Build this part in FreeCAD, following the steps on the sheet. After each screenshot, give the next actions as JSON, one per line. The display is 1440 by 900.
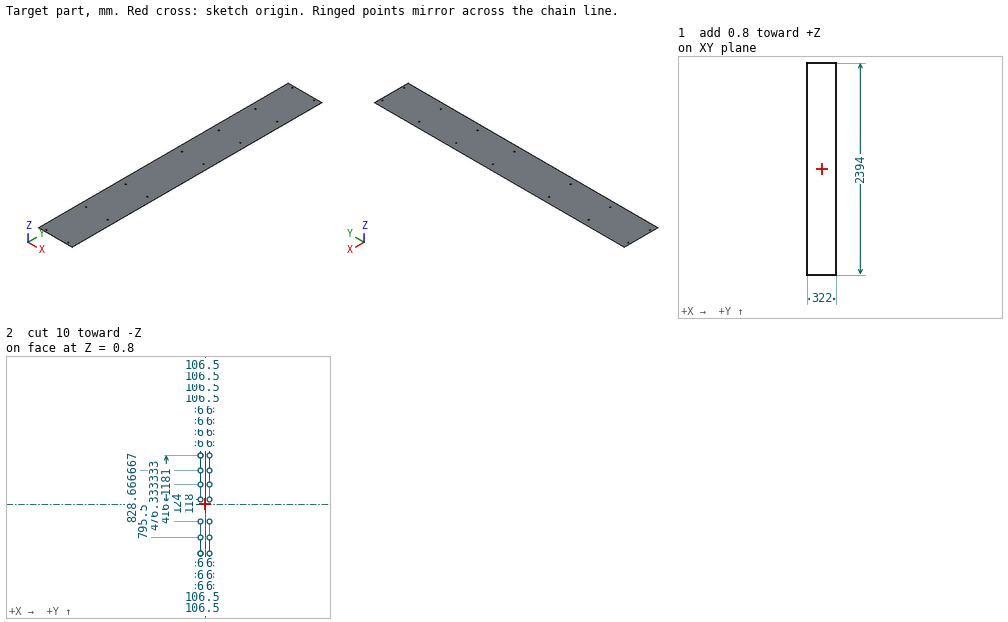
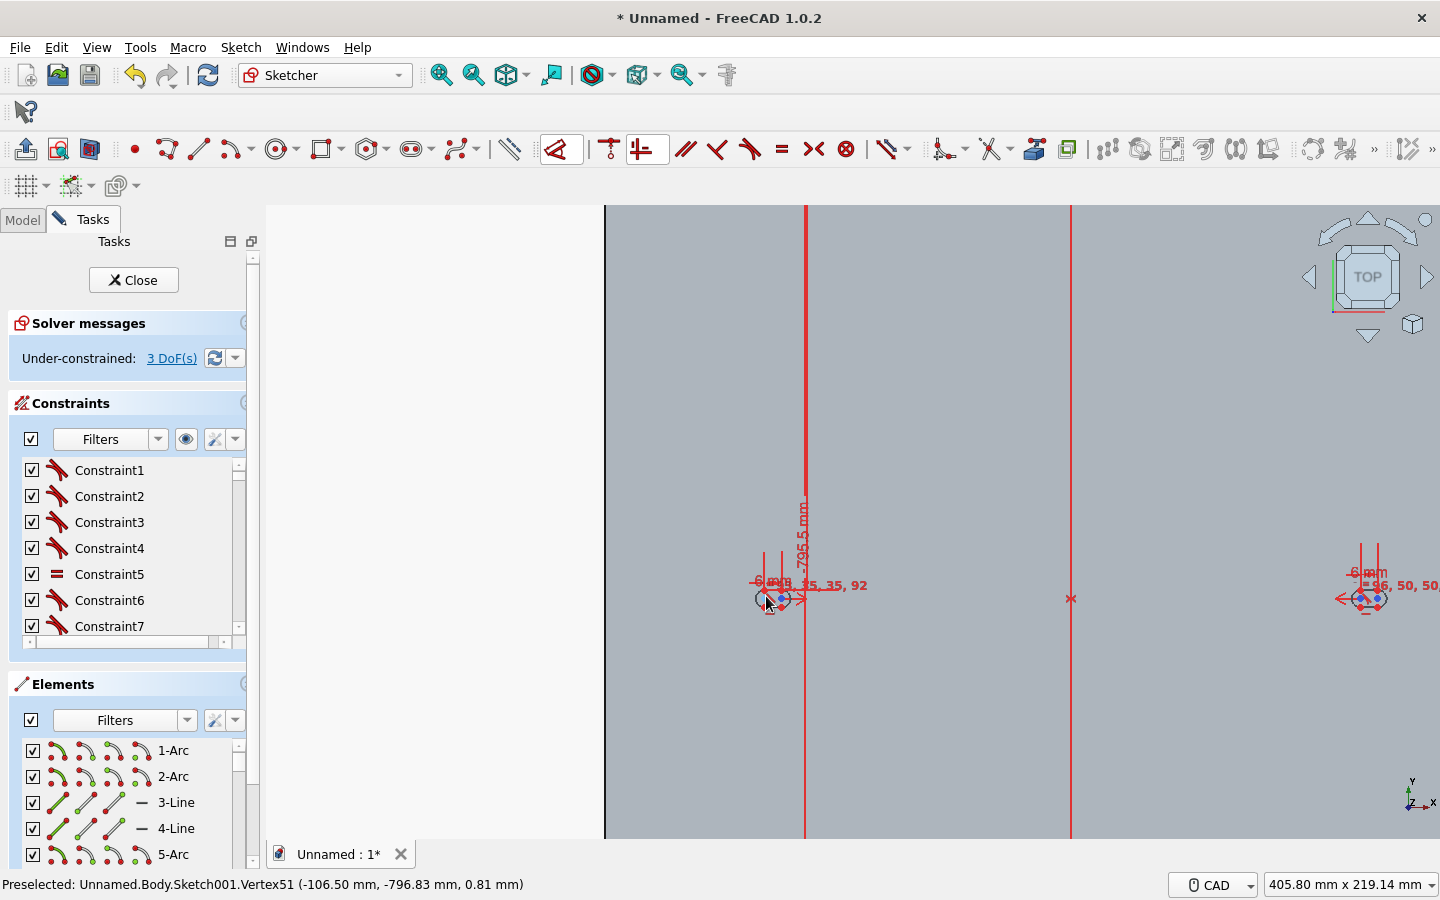
{"action": "left_click", "coordinate": [764, 590]}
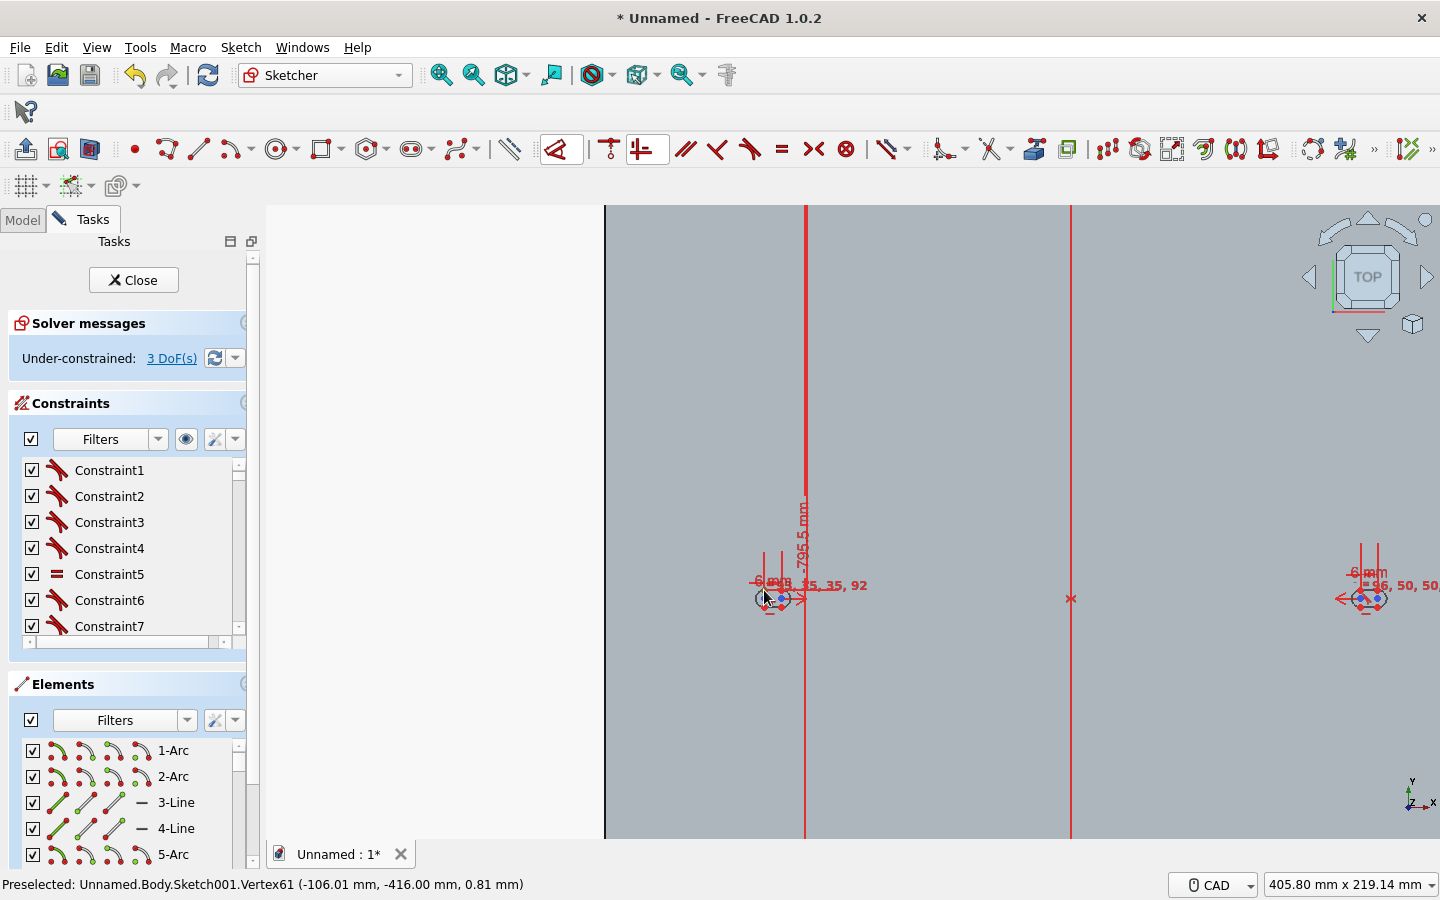
{"action": "key", "text": "l"}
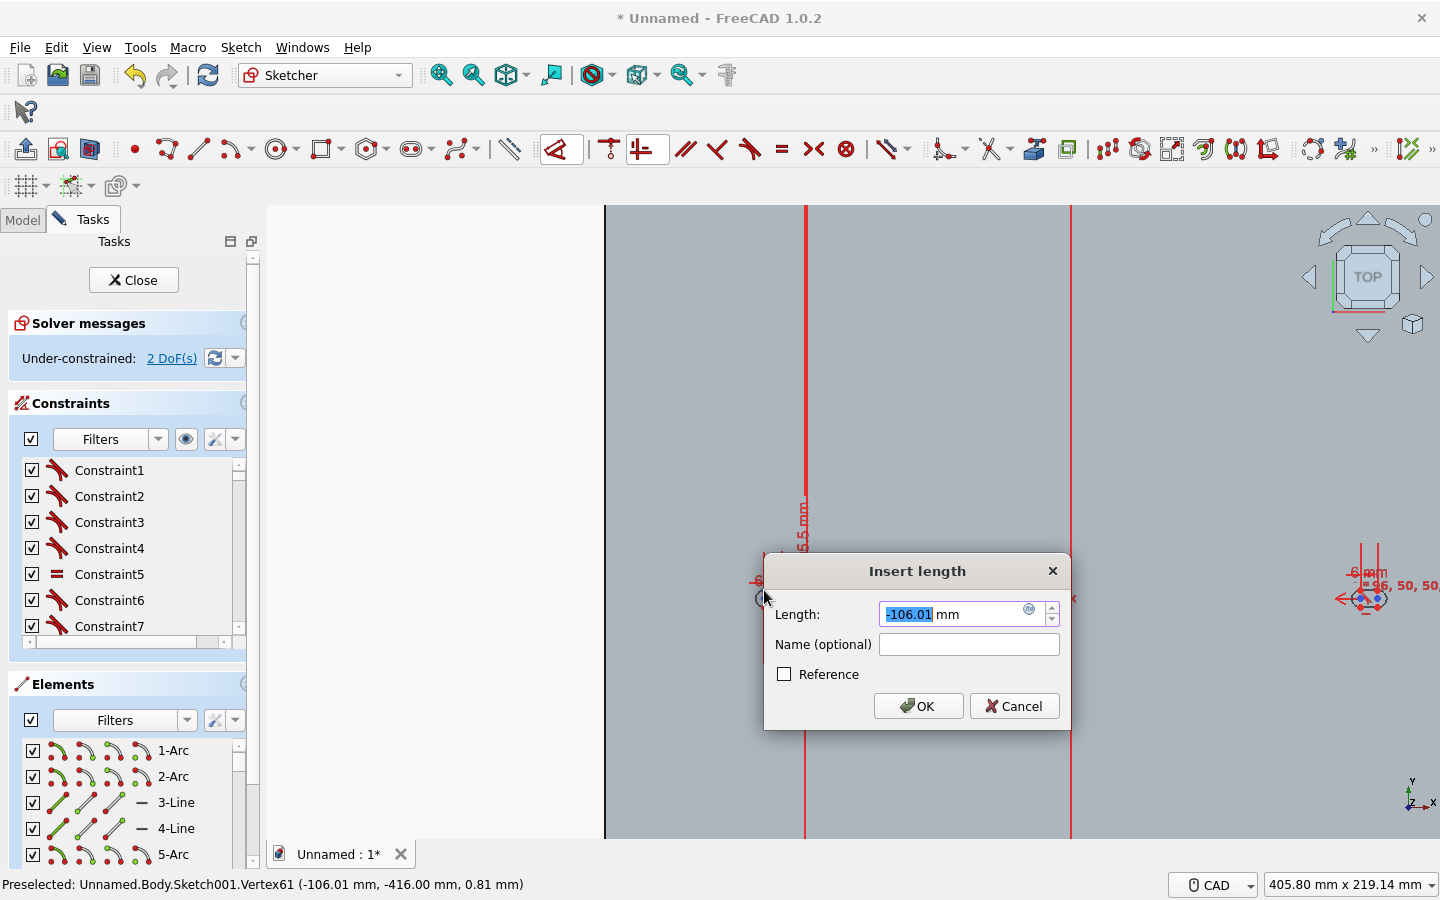
{"action": "type", "text": "-106.5"}
{"action": "key", "text": "Return"}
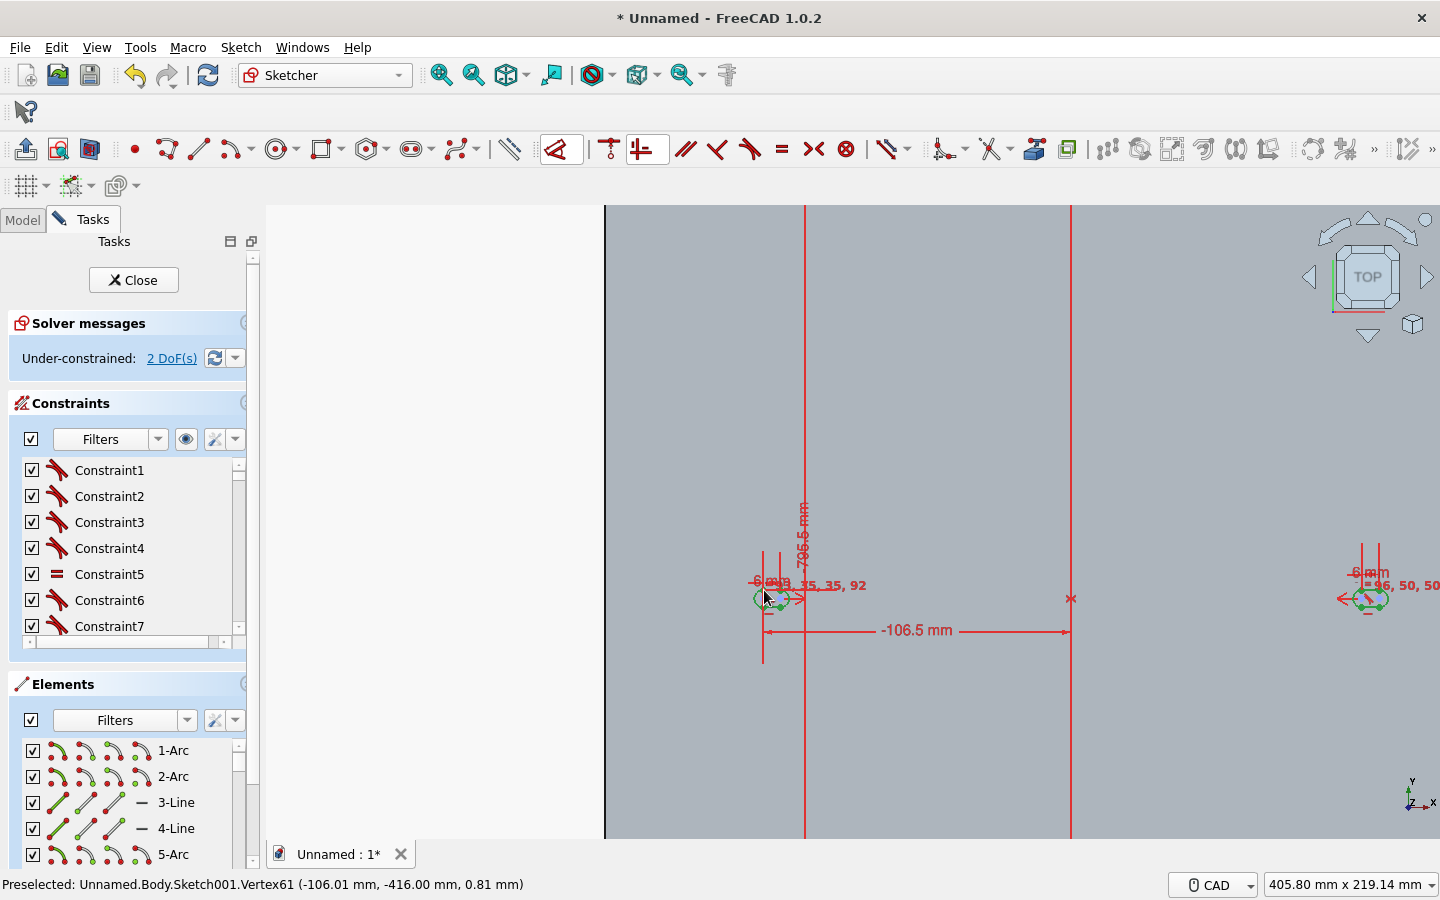
{"action": "scroll", "coordinate": [766, 596], "scroll_direction": "down", "scroll_amount": 14}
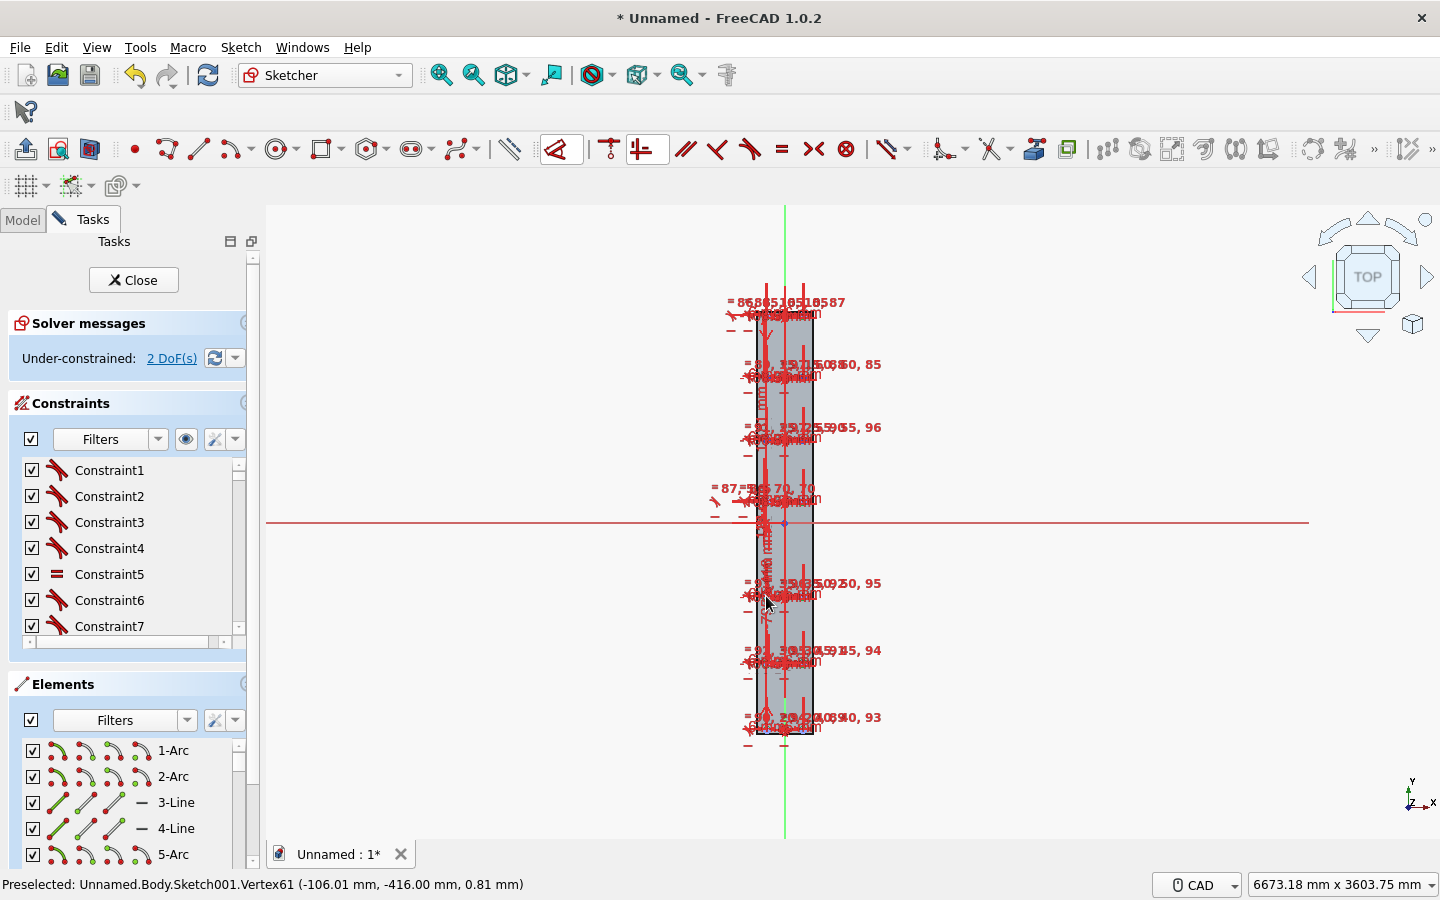
{"action": "scroll", "coordinate": [766, 377], "scroll_direction": "up", "scroll_amount": 14}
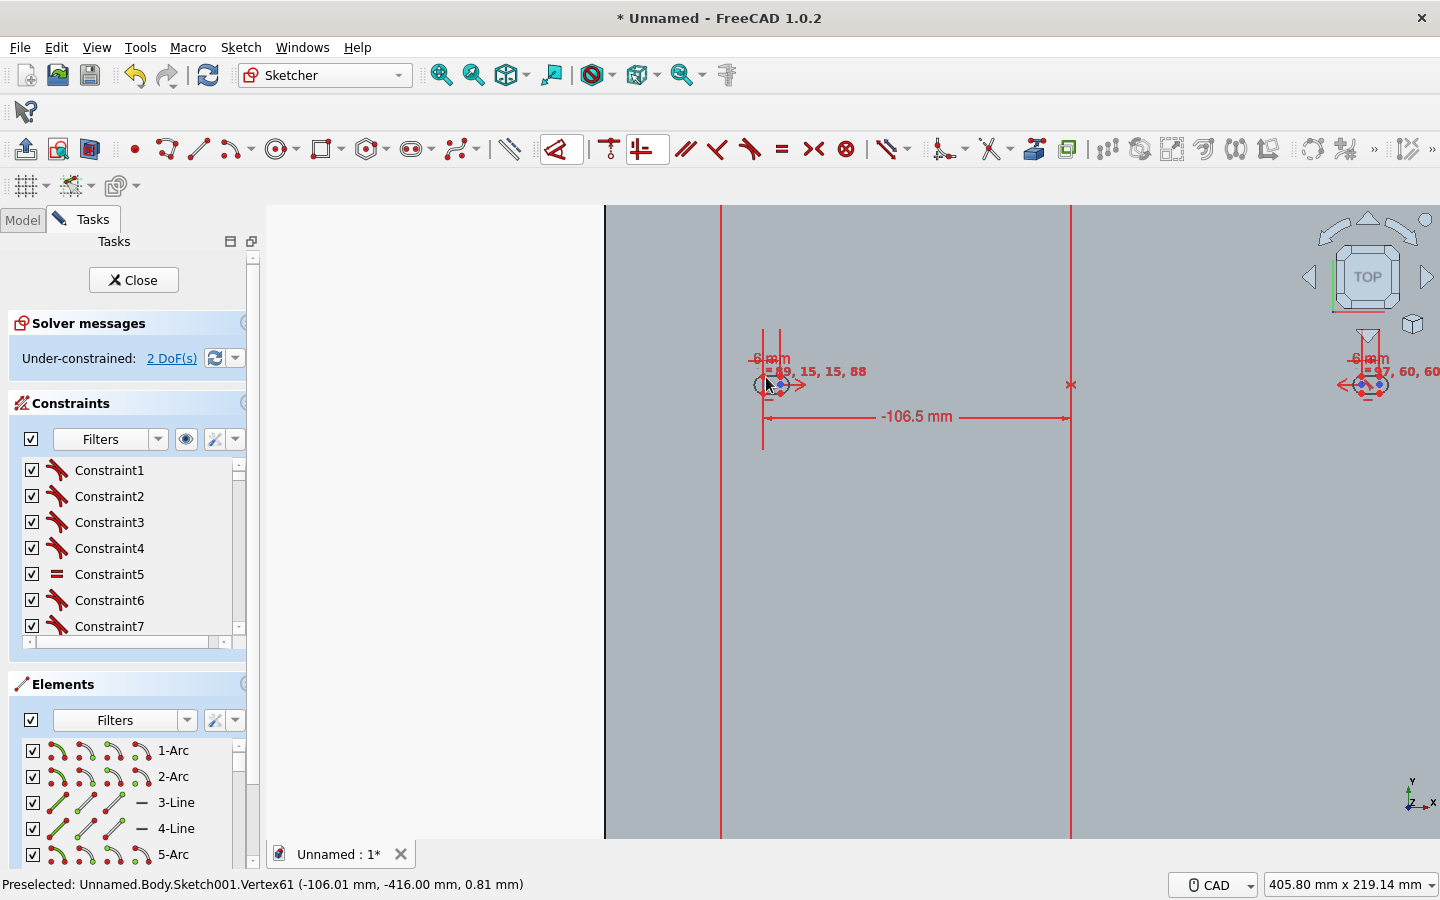
{"action": "left_click", "coordinate": [763, 376]}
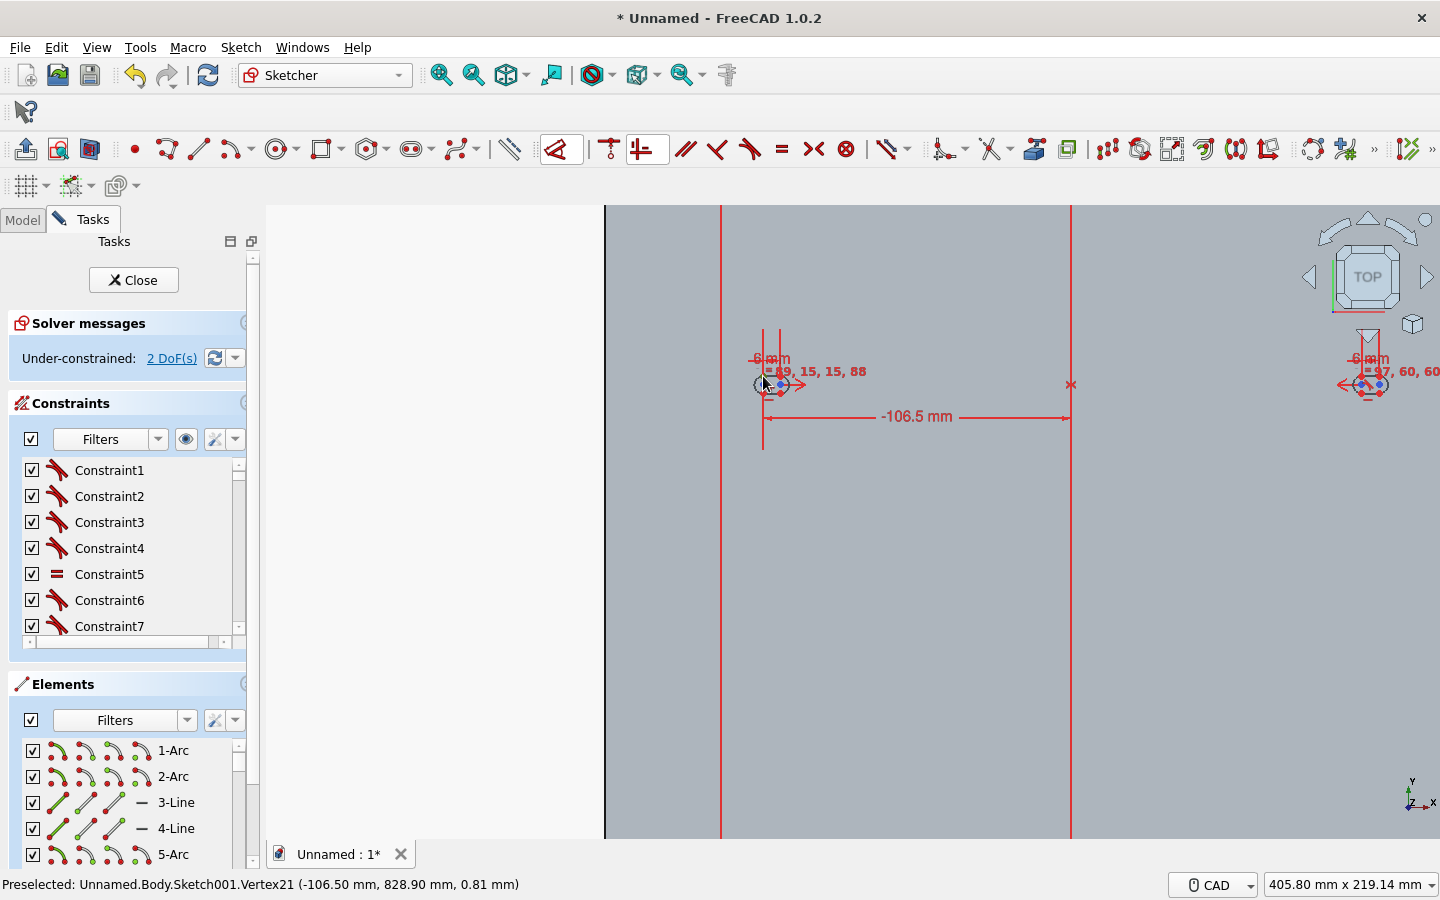
{"action": "key", "text": "i"}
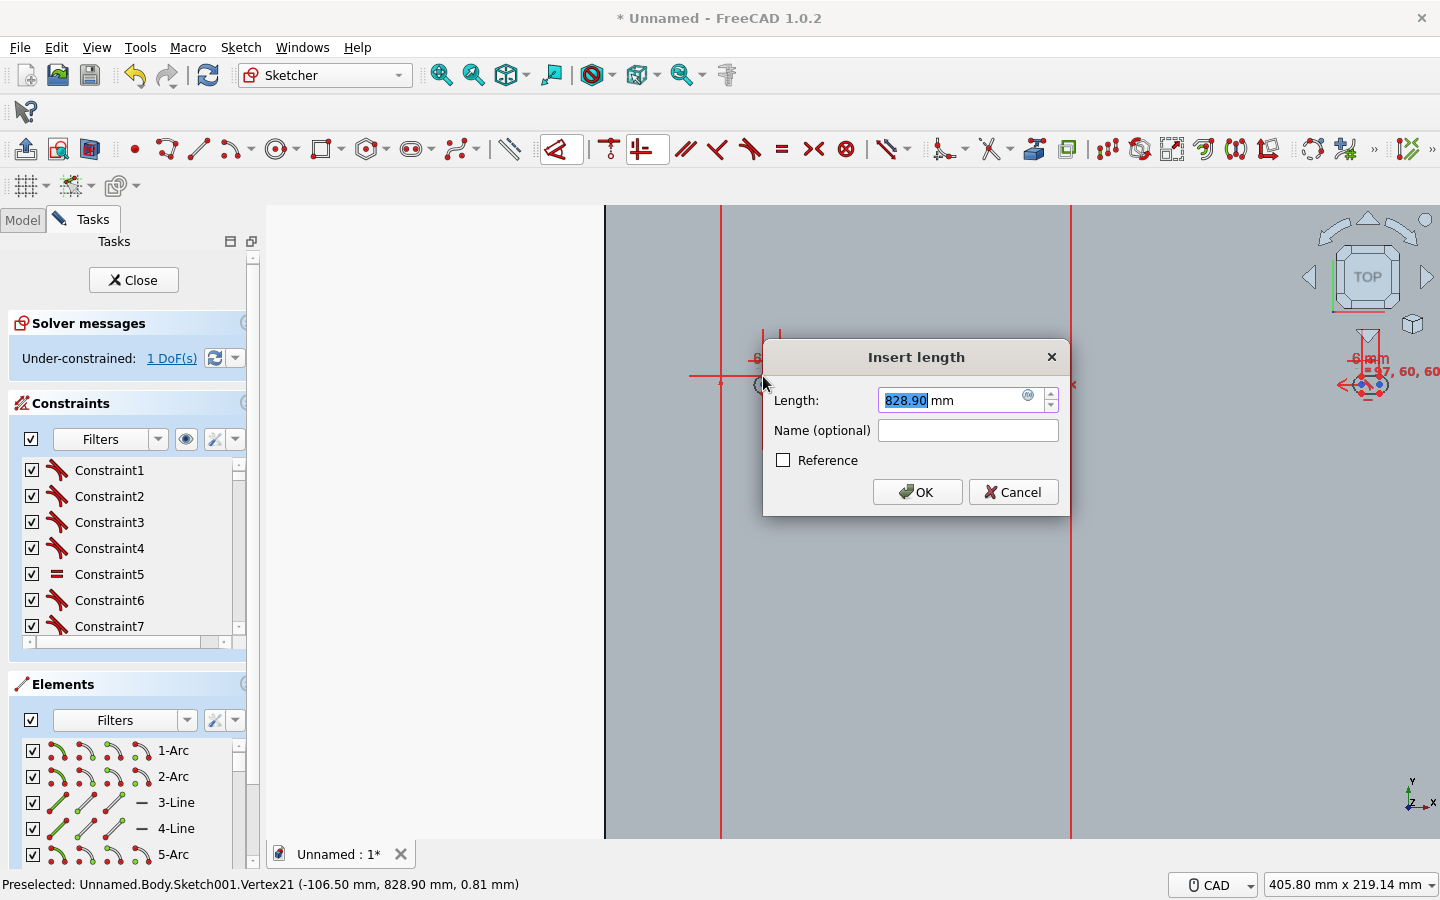
{"action": "type", "text": "828.666667"}
{"action": "key", "text": "Return"}